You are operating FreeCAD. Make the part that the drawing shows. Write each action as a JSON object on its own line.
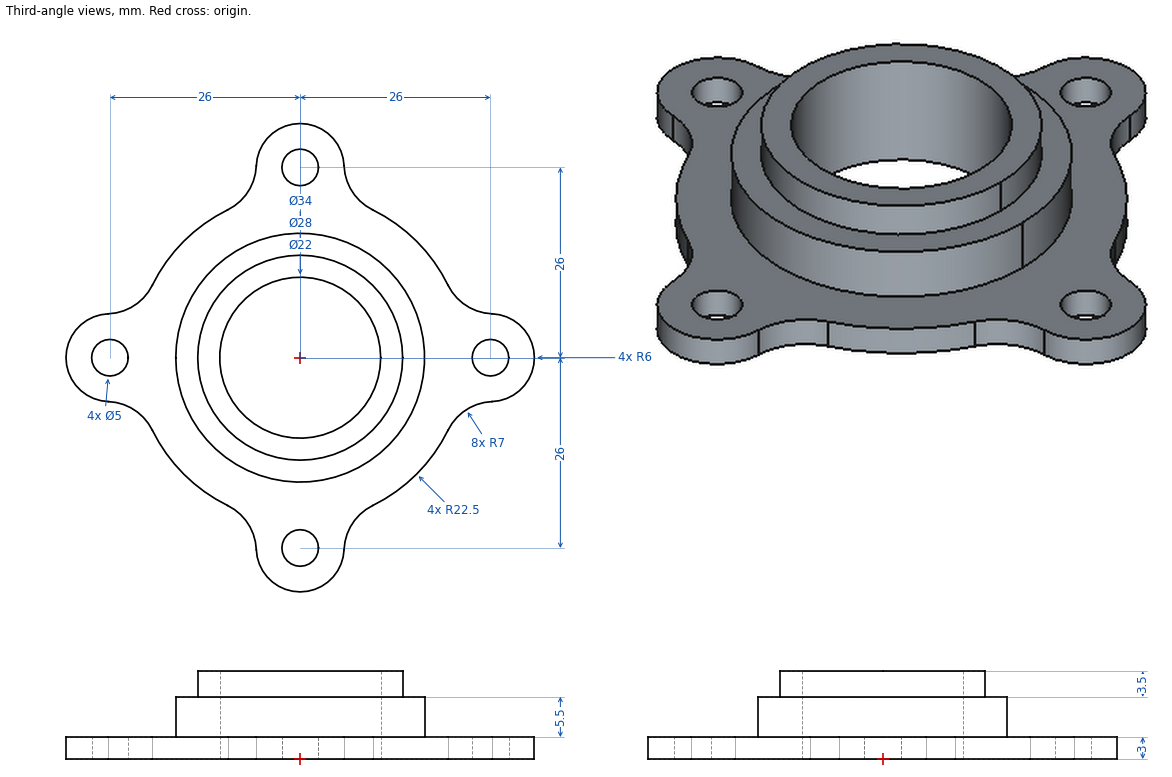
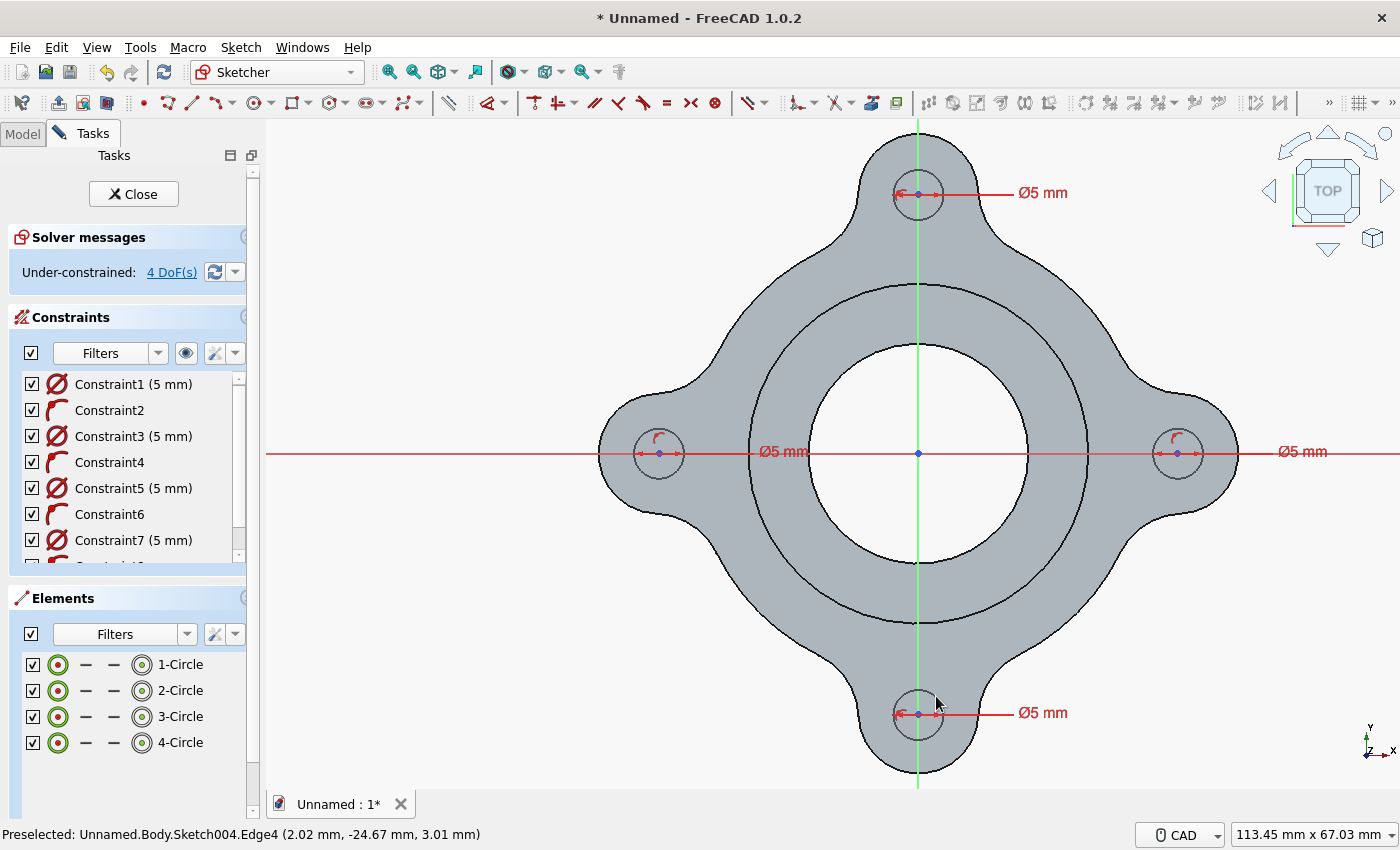
{"action": "left_click", "coordinate": [488, 104]}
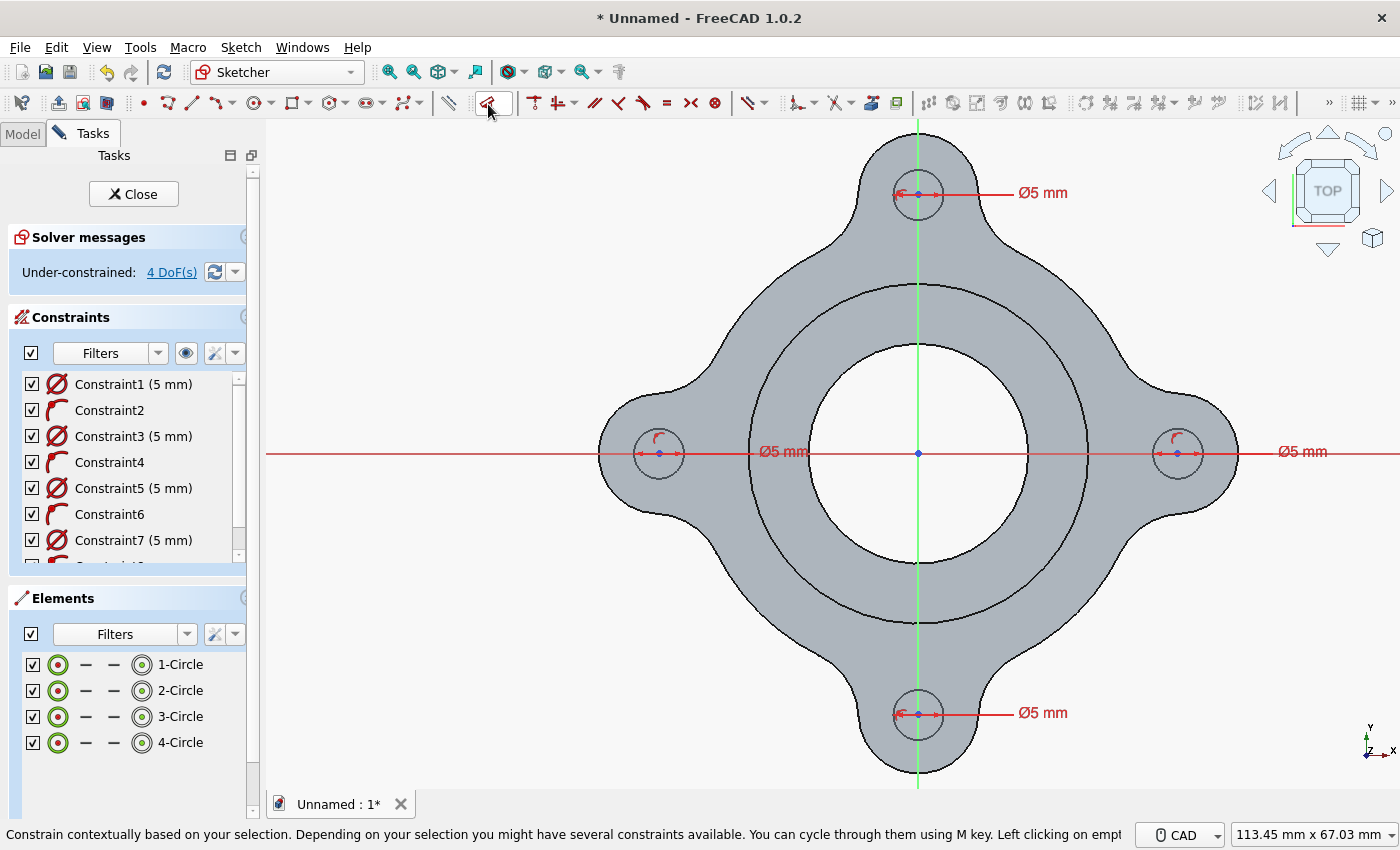
{"action": "left_click", "coordinate": [659, 454]}
{"action": "left_click", "coordinate": [789, 488]}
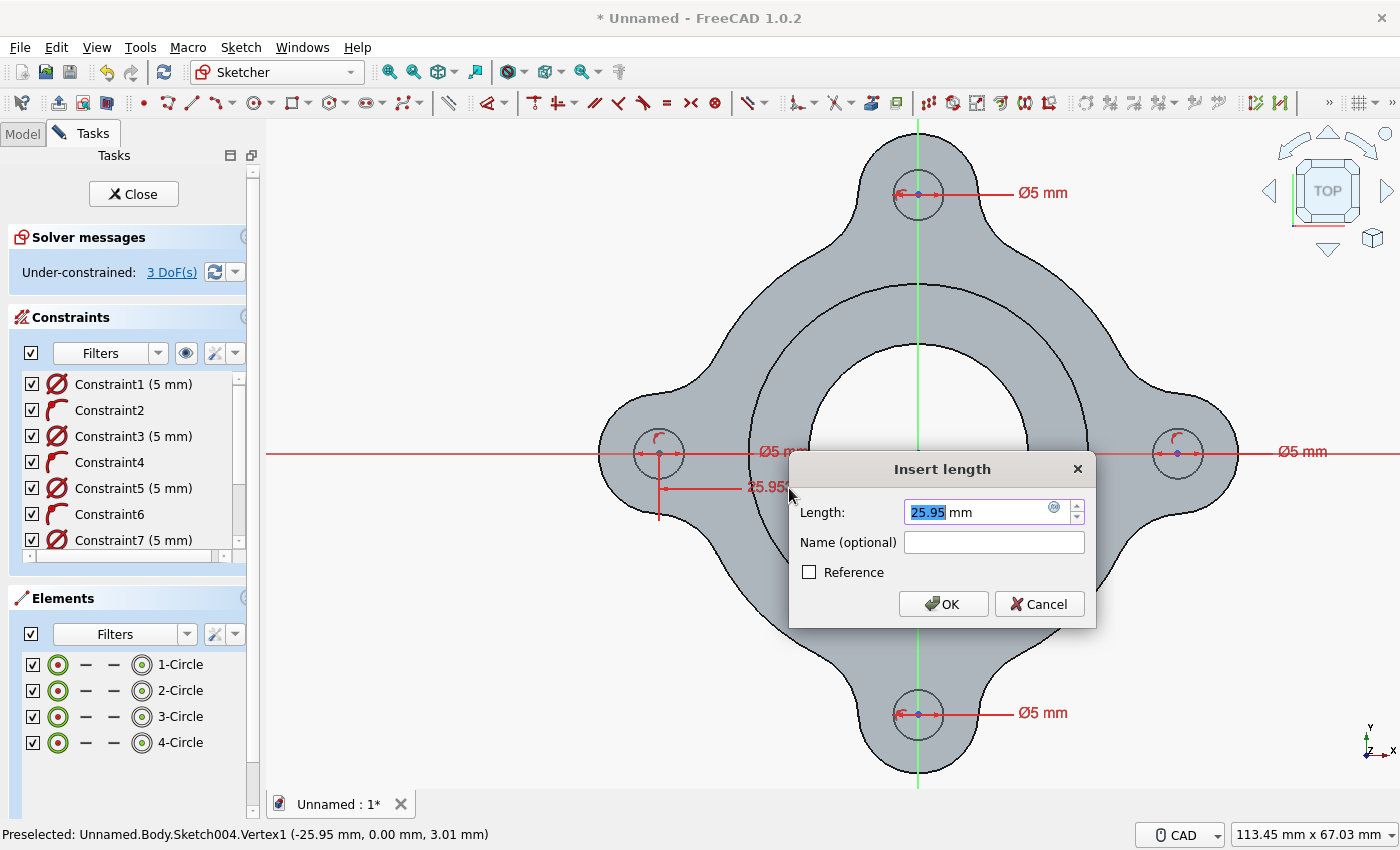
{"action": "type", "text": "26"}
{"action": "key", "text": "Return"}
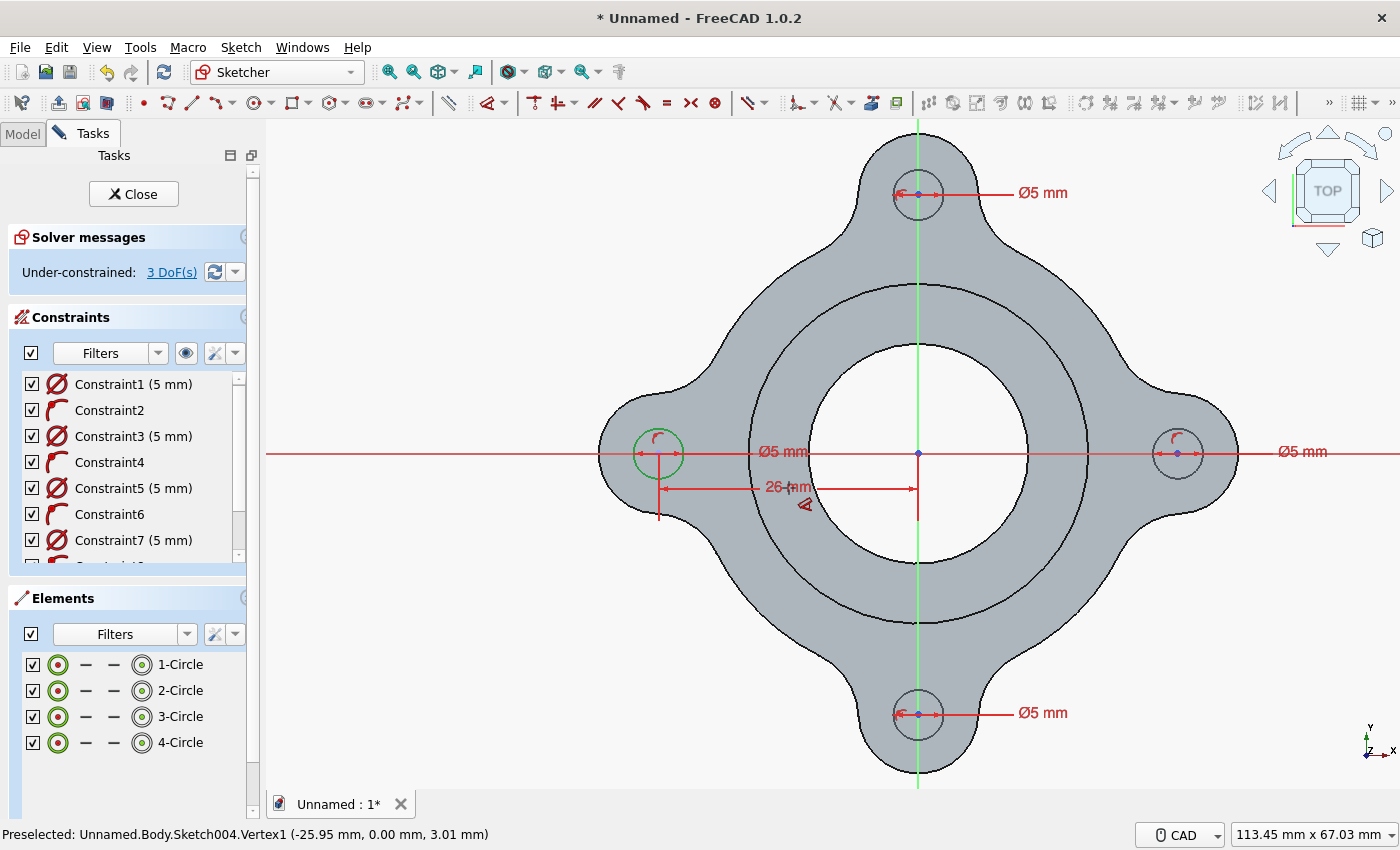
{"action": "left_click", "coordinate": [918, 195]}
{"action": "left_click", "coordinate": [952, 324]}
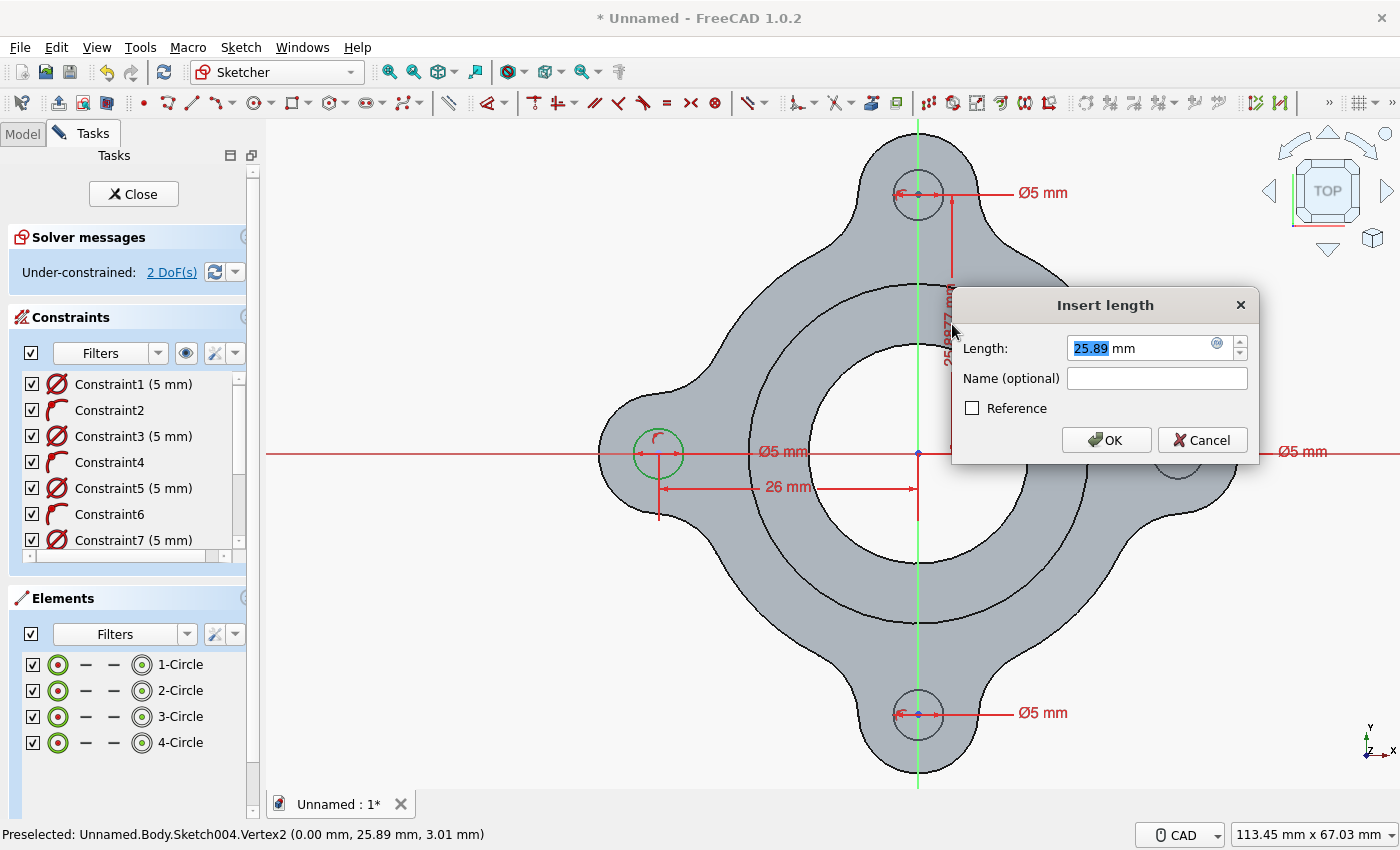
{"action": "type", "text": "26"}
{"action": "key", "text": "Return"}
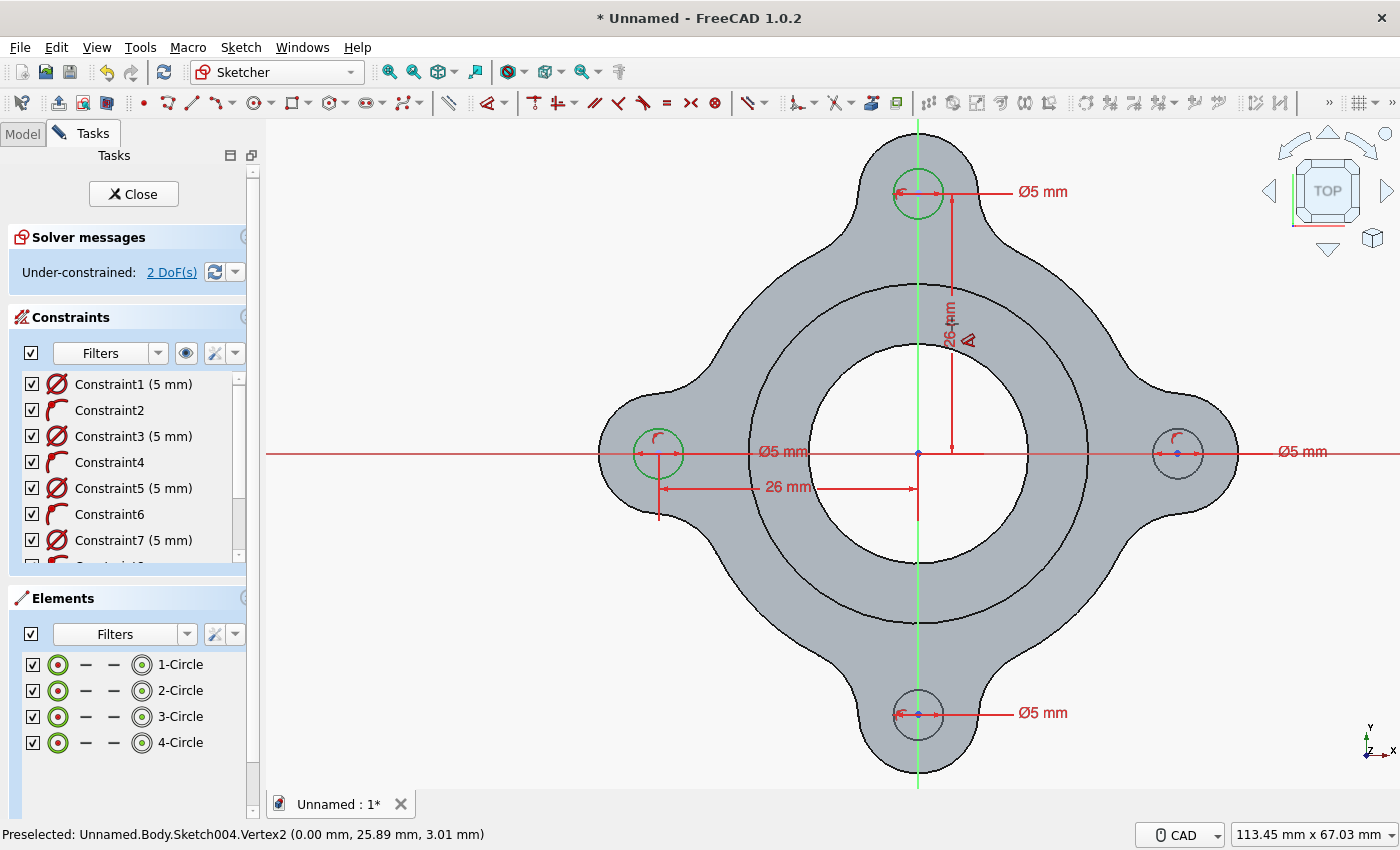
{"action": "left_click", "coordinate": [1178, 454]}
{"action": "left_click", "coordinate": [1048, 488]}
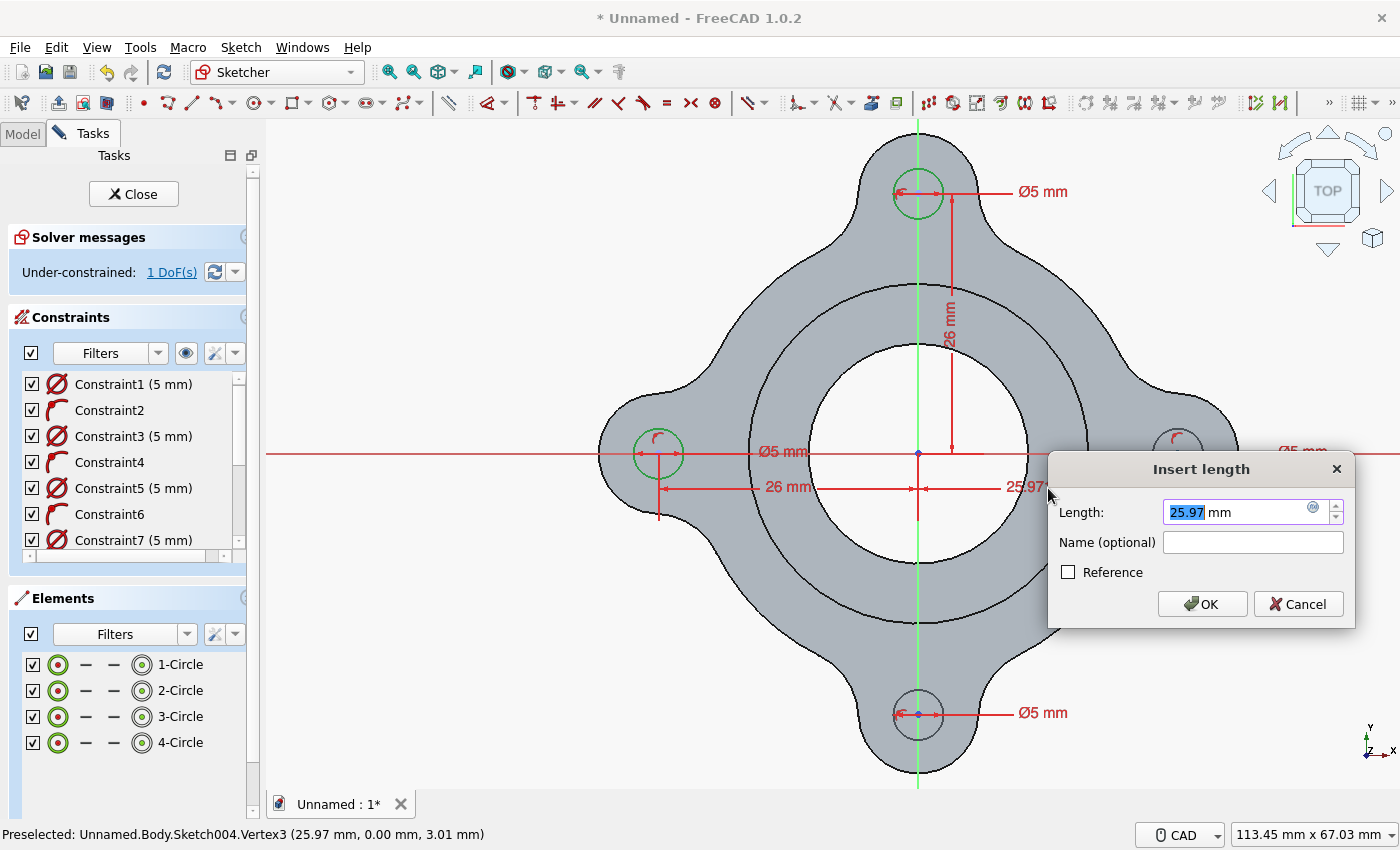
{"action": "type", "text": "26"}
{"action": "key", "text": "Return"}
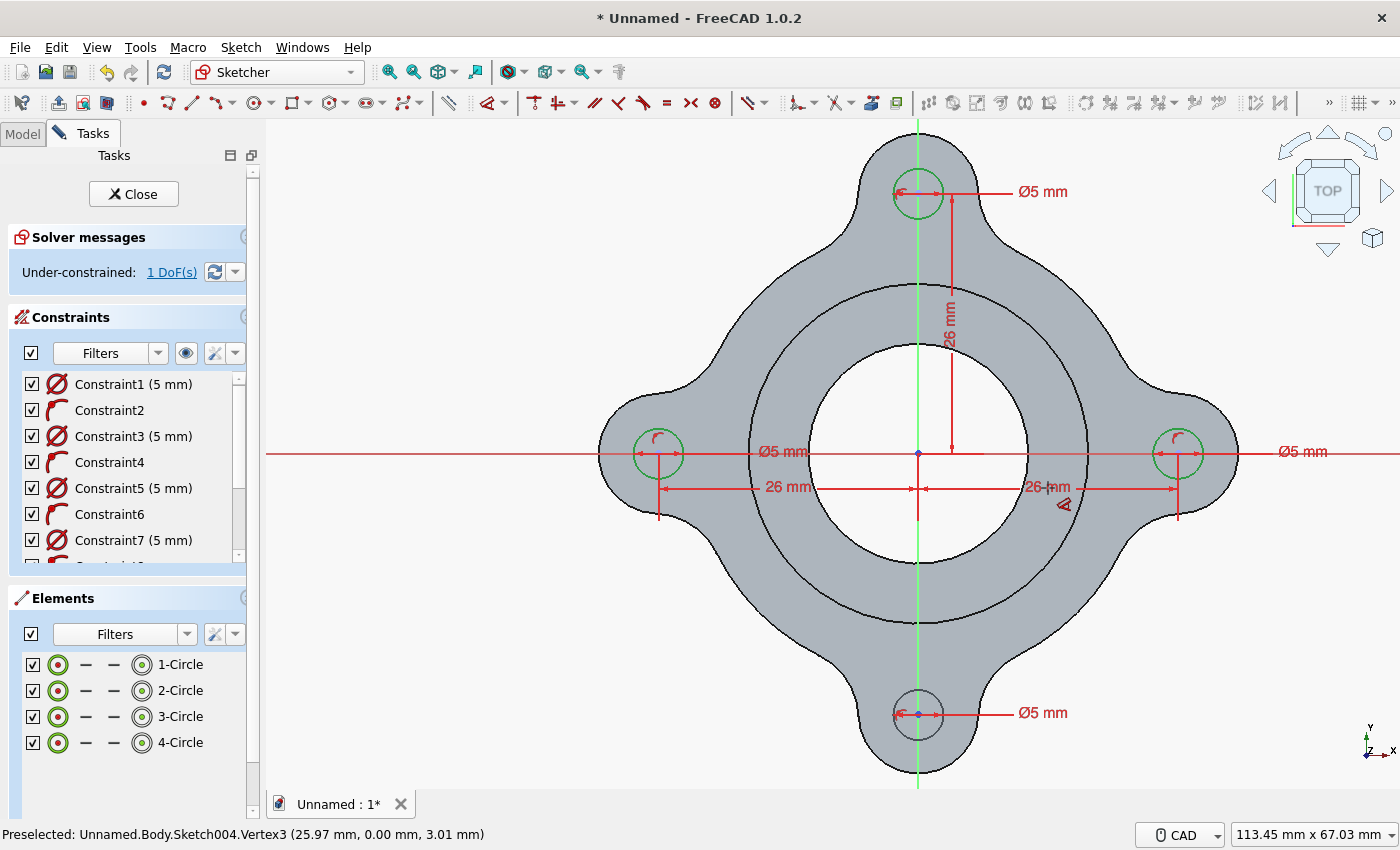
{"action": "left_click", "coordinate": [918, 715]}
{"action": "left_click", "coordinate": [952, 584]}